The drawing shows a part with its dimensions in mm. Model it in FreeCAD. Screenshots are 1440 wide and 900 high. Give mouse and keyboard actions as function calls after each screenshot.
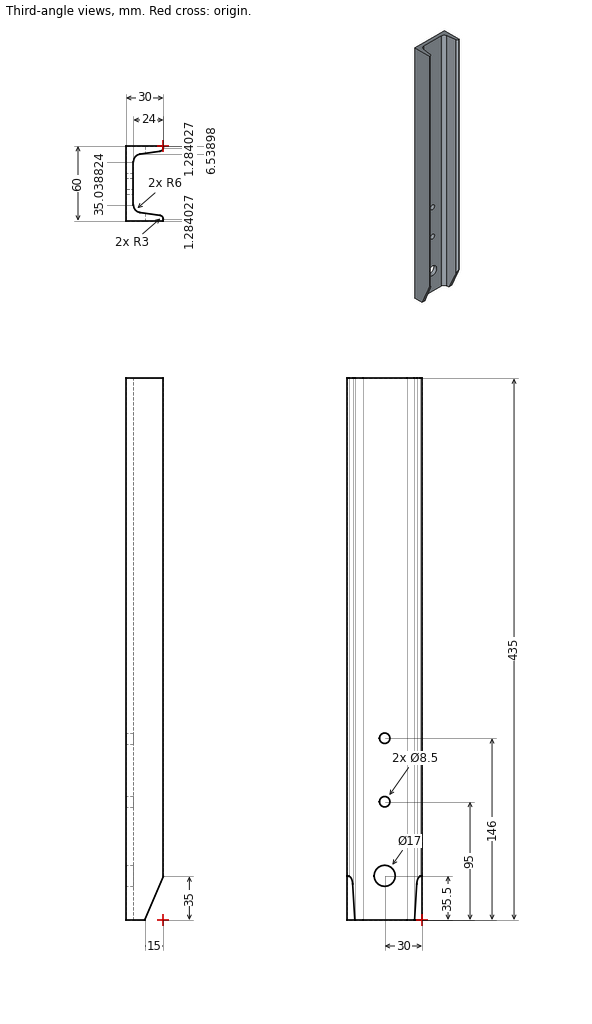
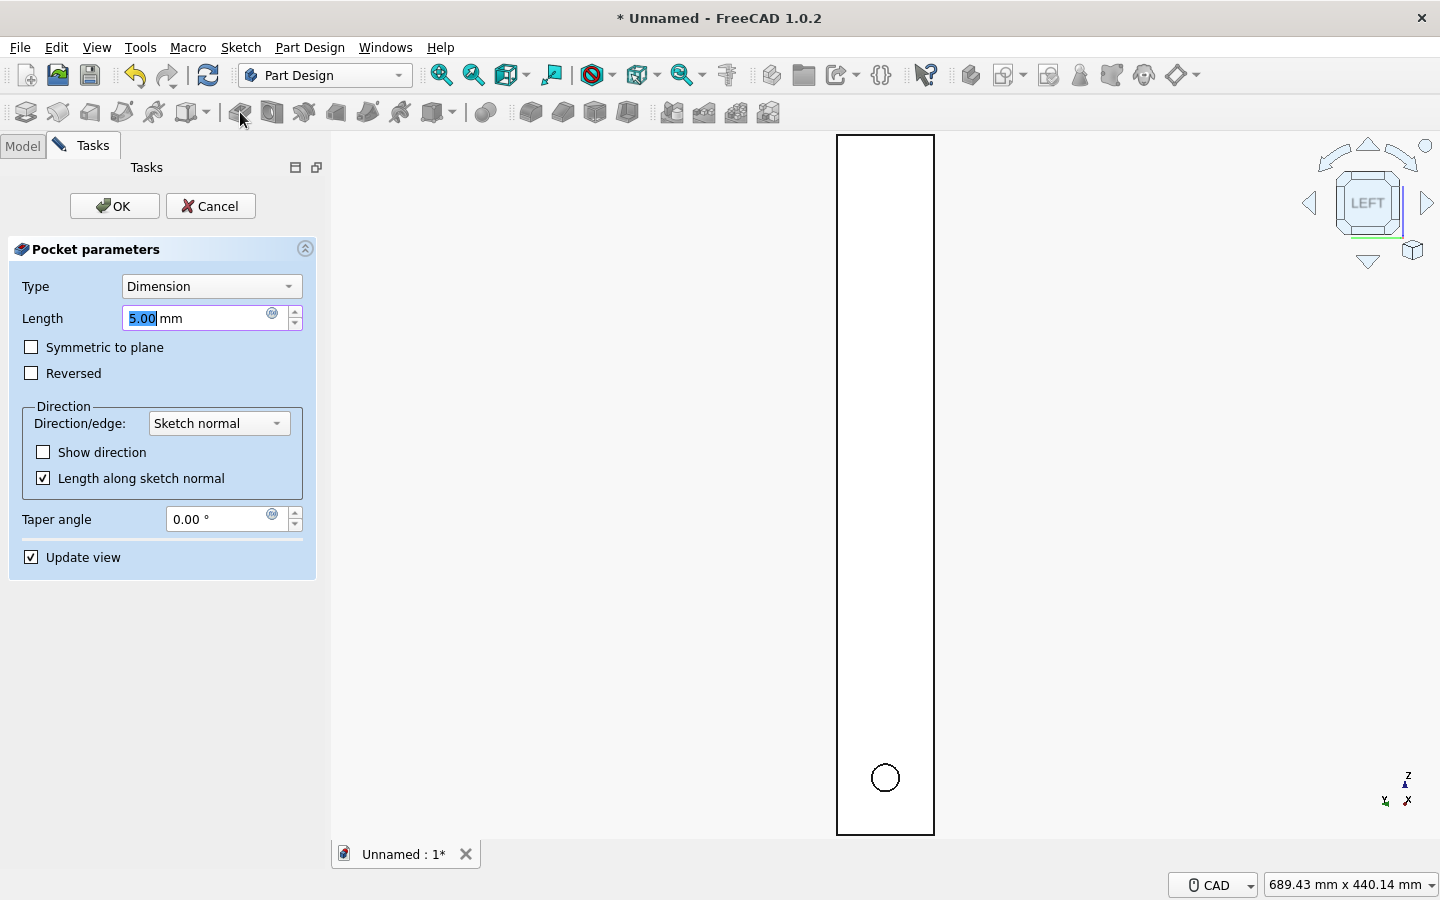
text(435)
key(Tab)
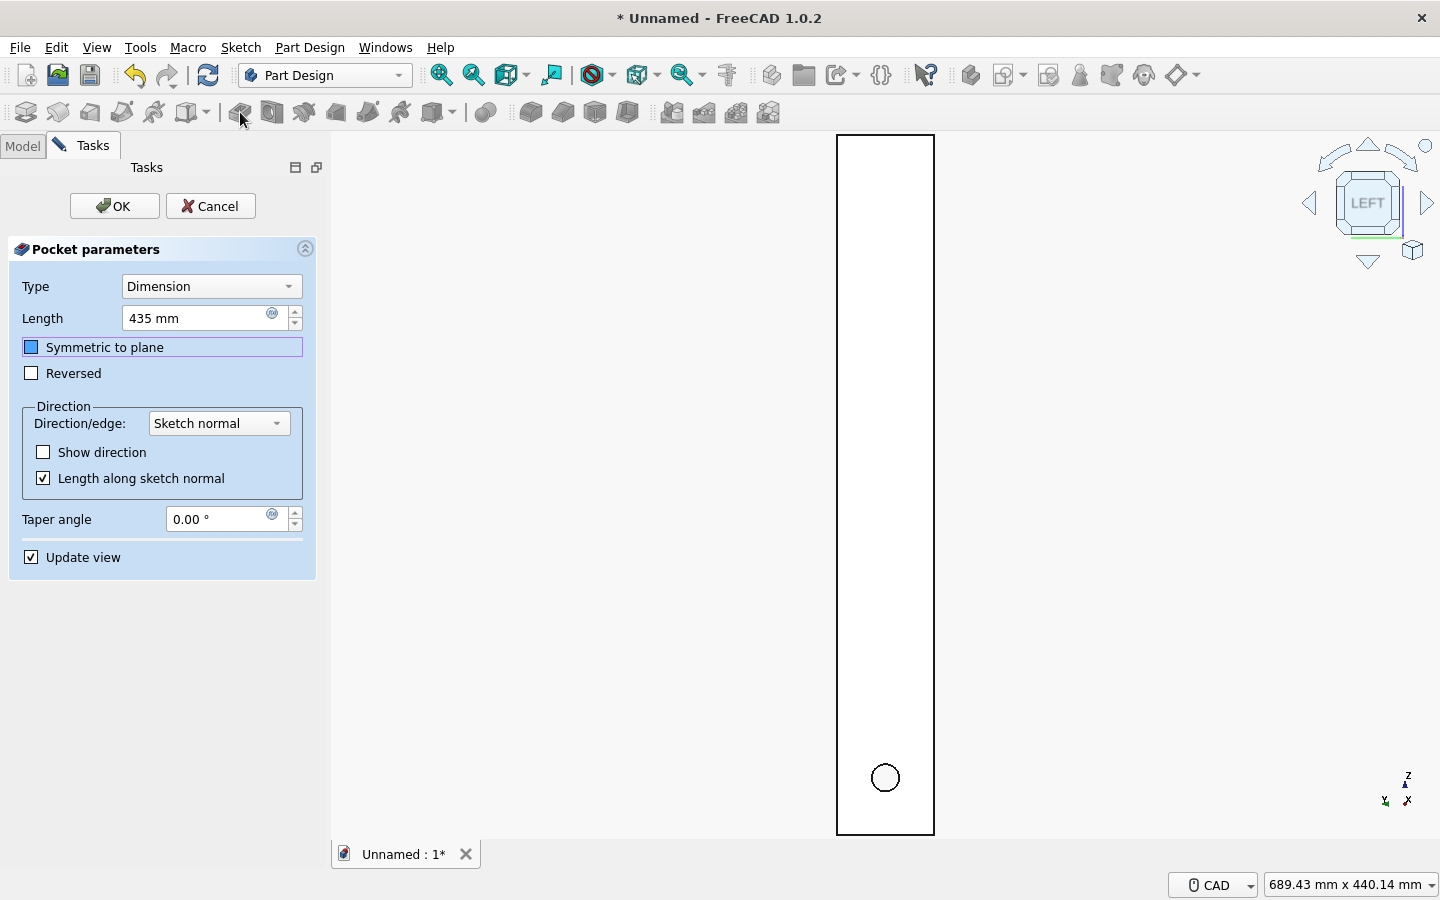
click(115, 206)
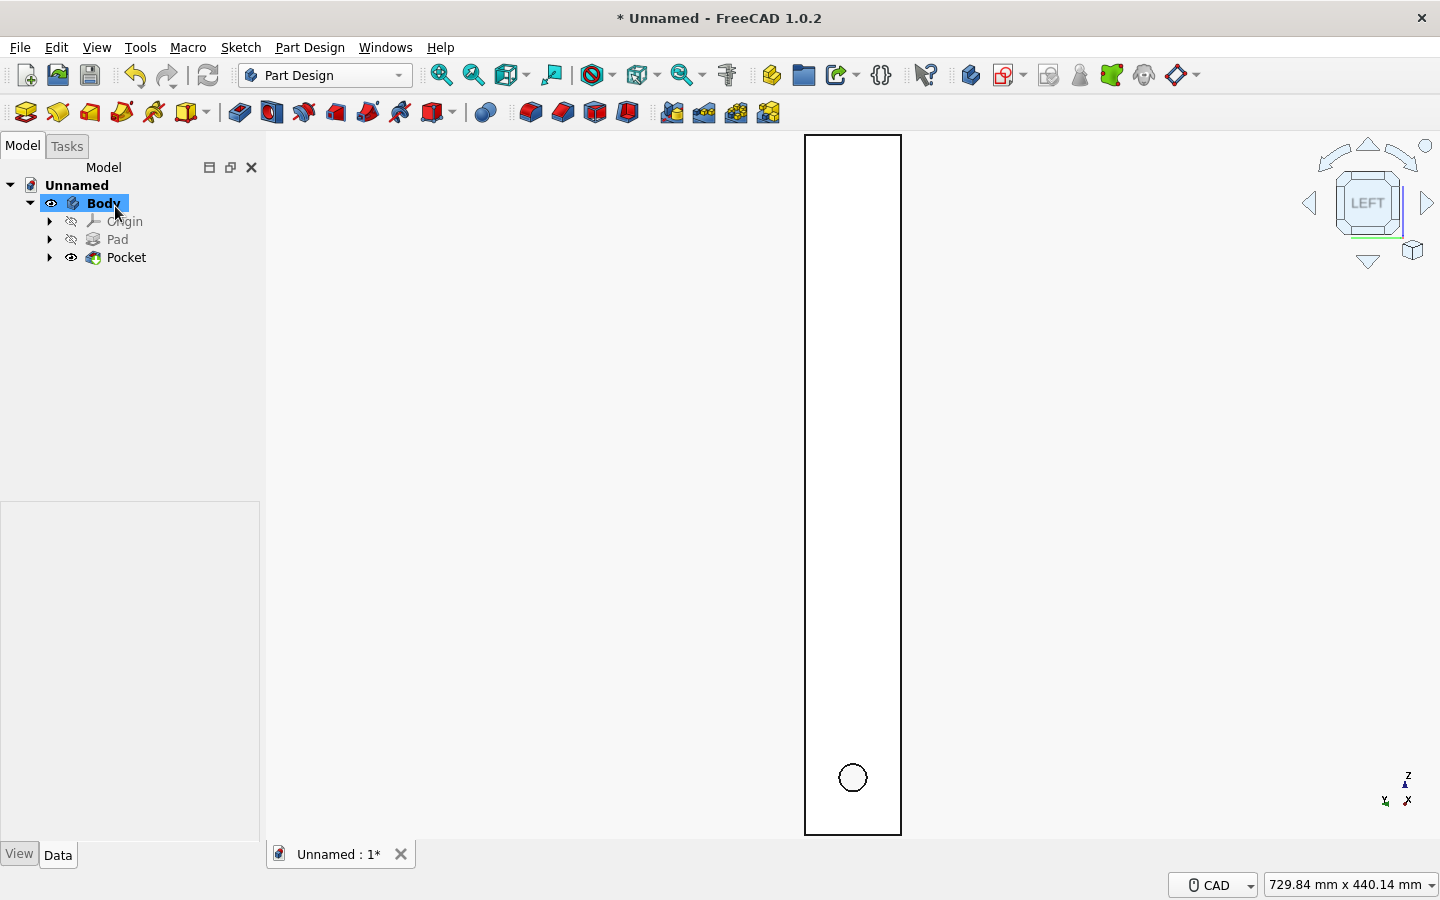
click(1004, 76)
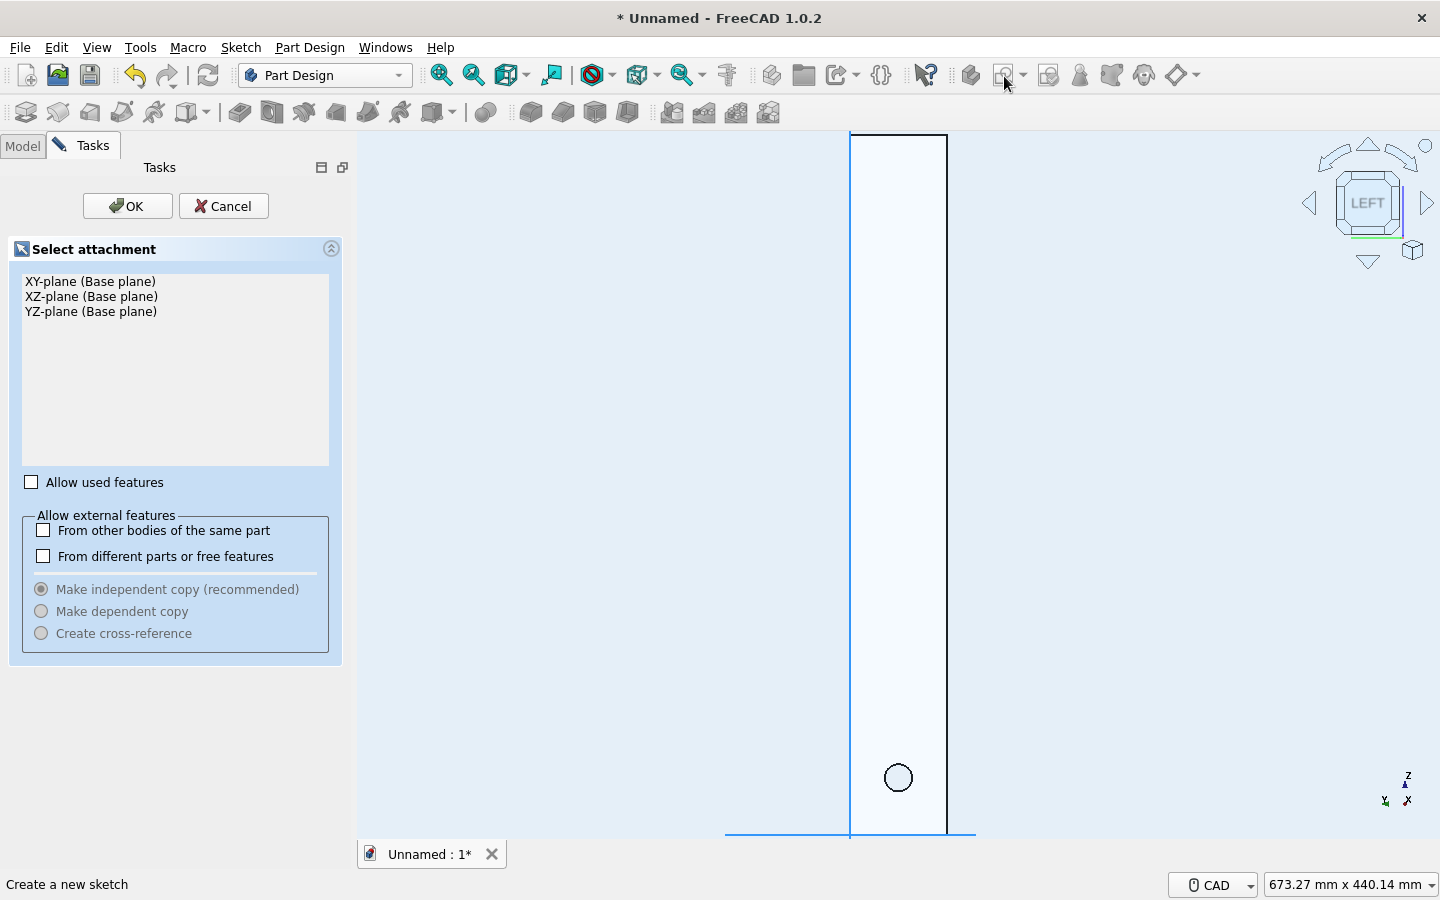
click(82, 296)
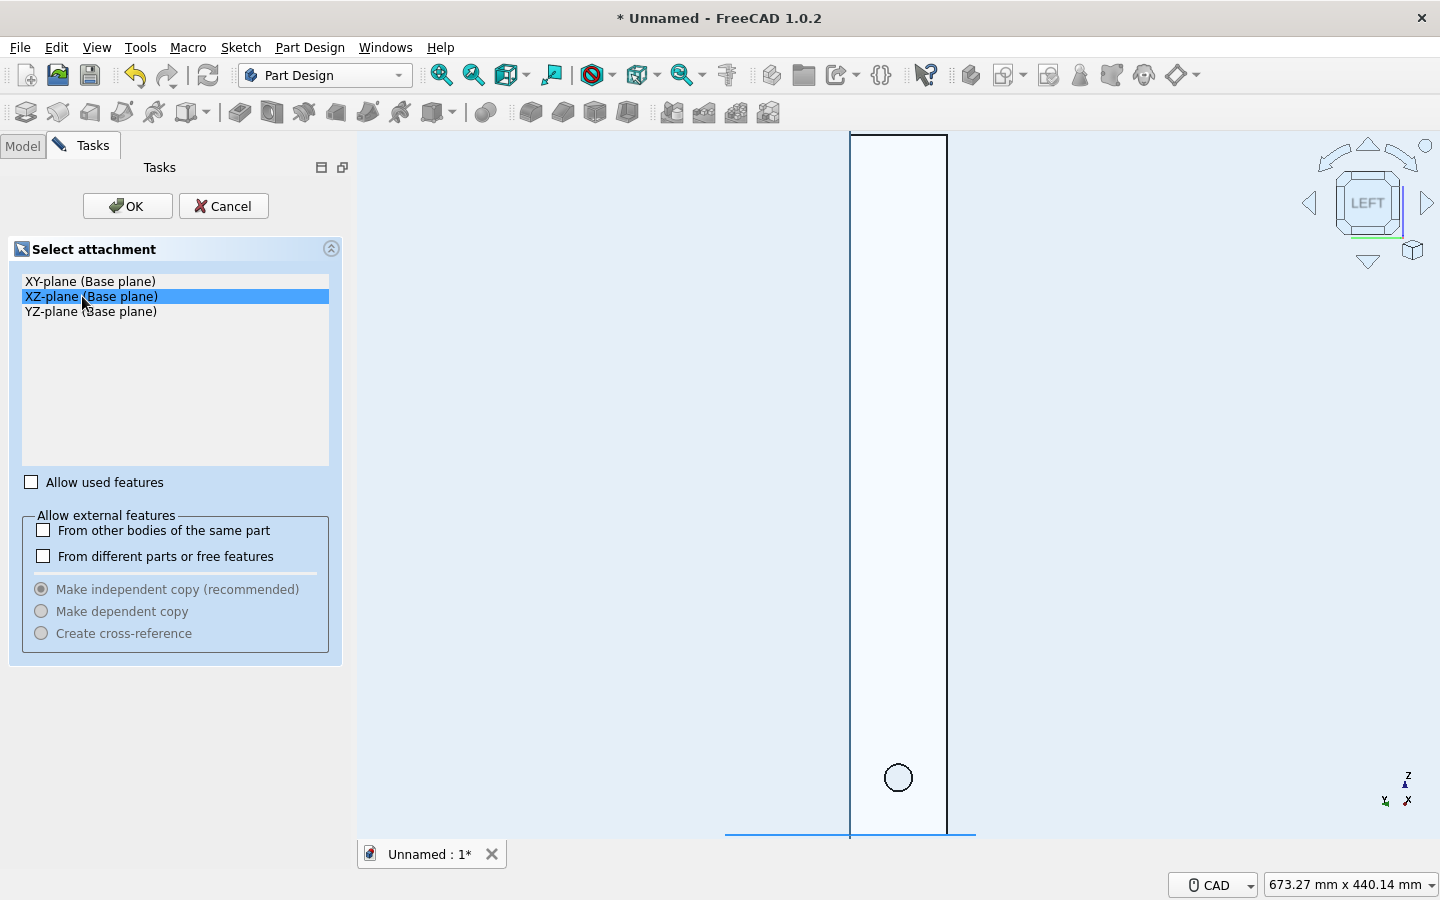
click(128, 206)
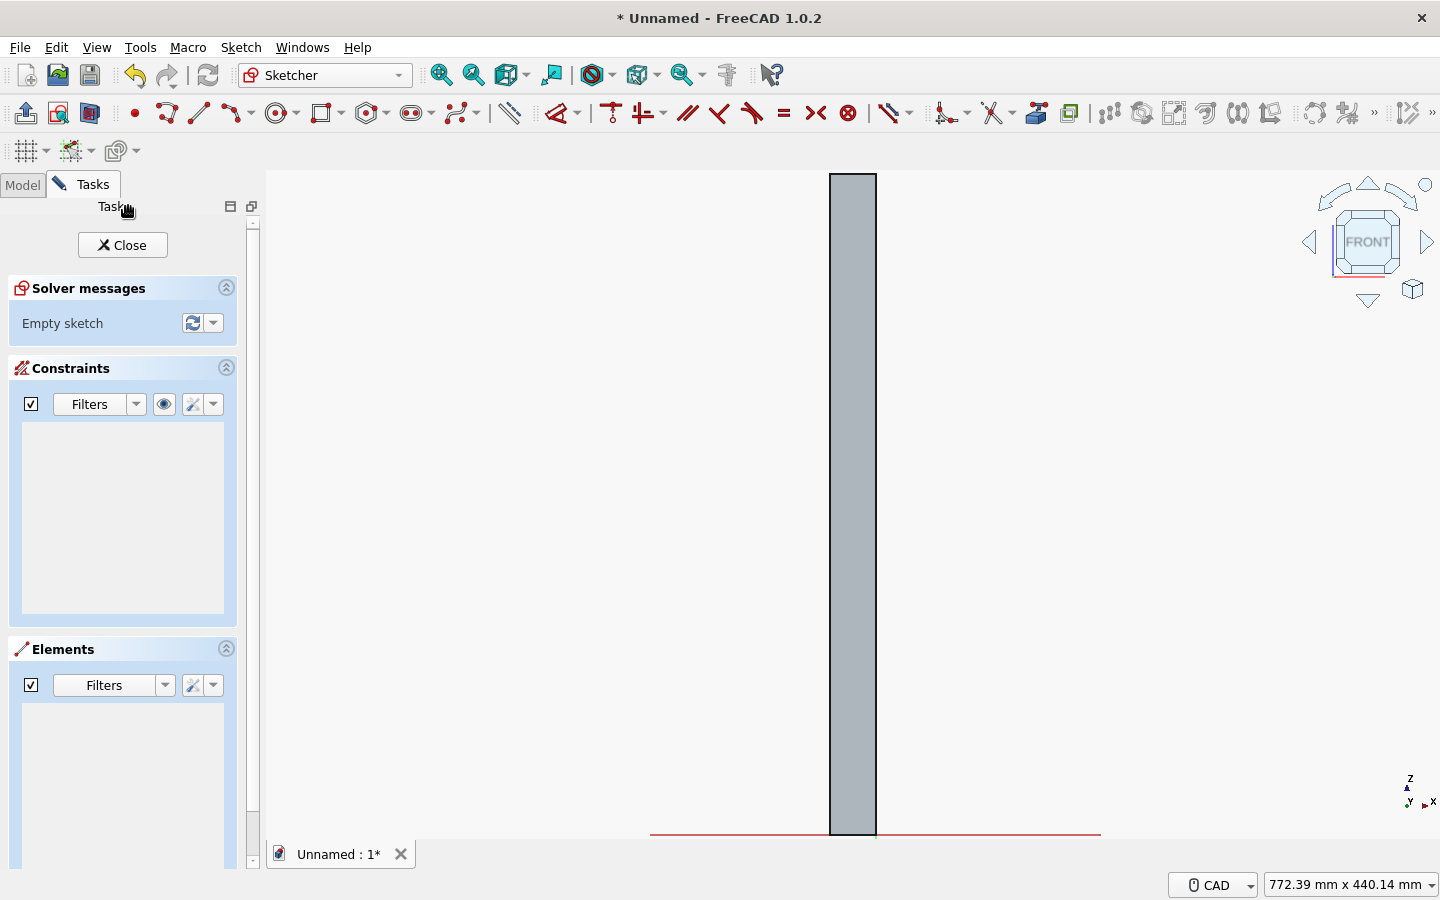
key(q)
key(s)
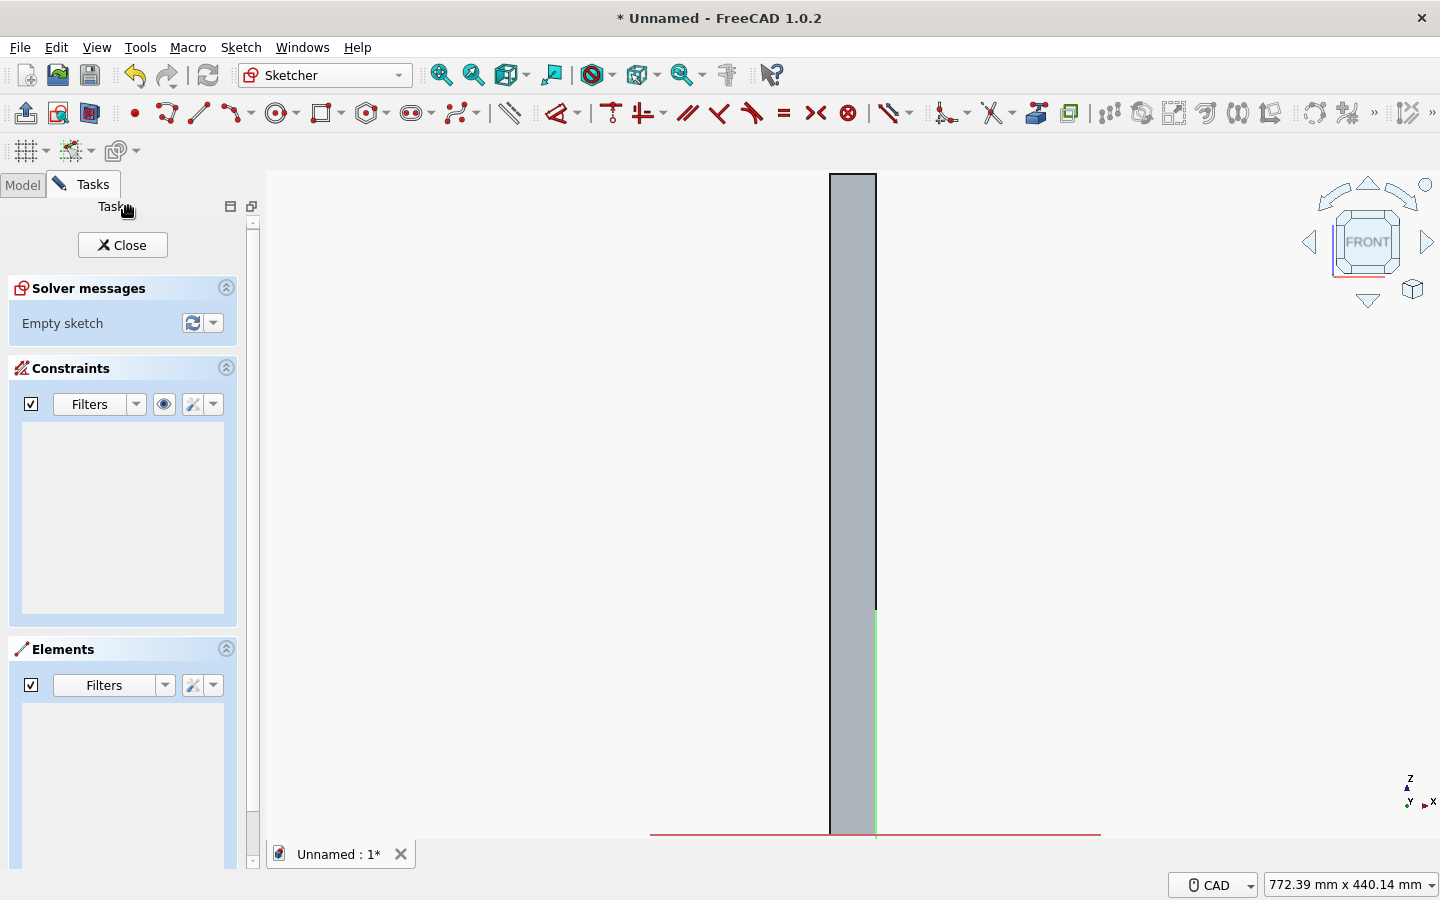
scroll(784, 504, down, 5)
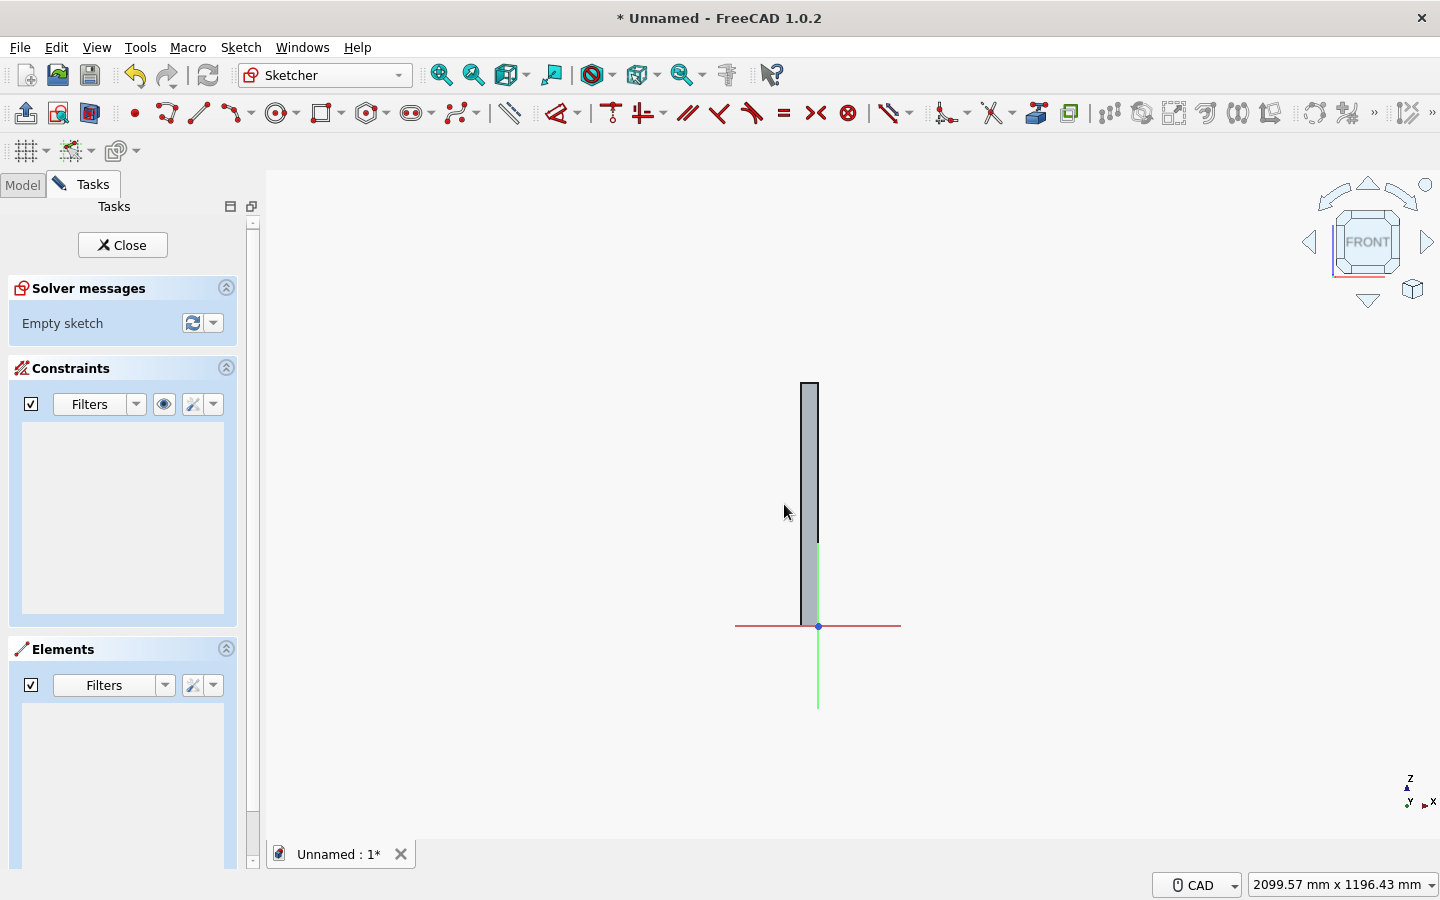
scroll(815, 622, up, 15)